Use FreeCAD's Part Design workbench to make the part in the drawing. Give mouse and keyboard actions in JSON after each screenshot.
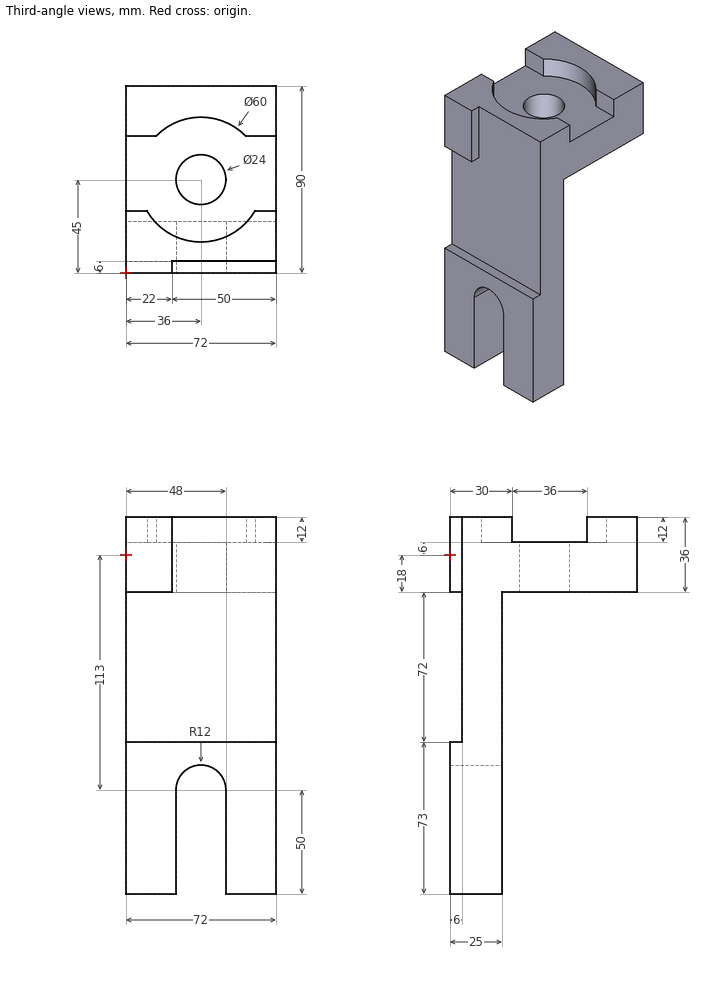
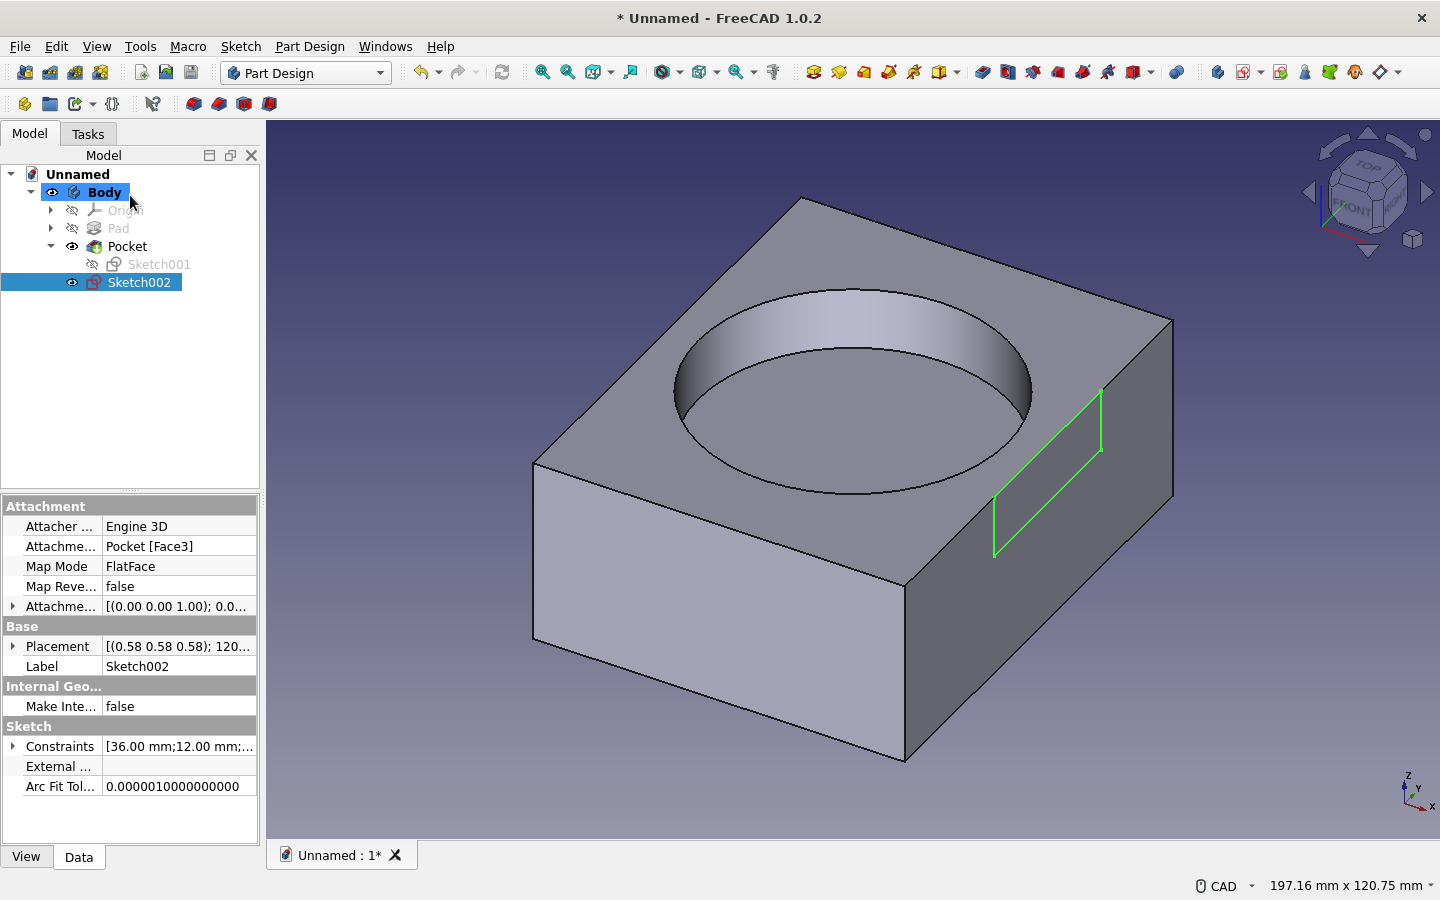
{"action": "left_click", "coordinate": [983, 72]}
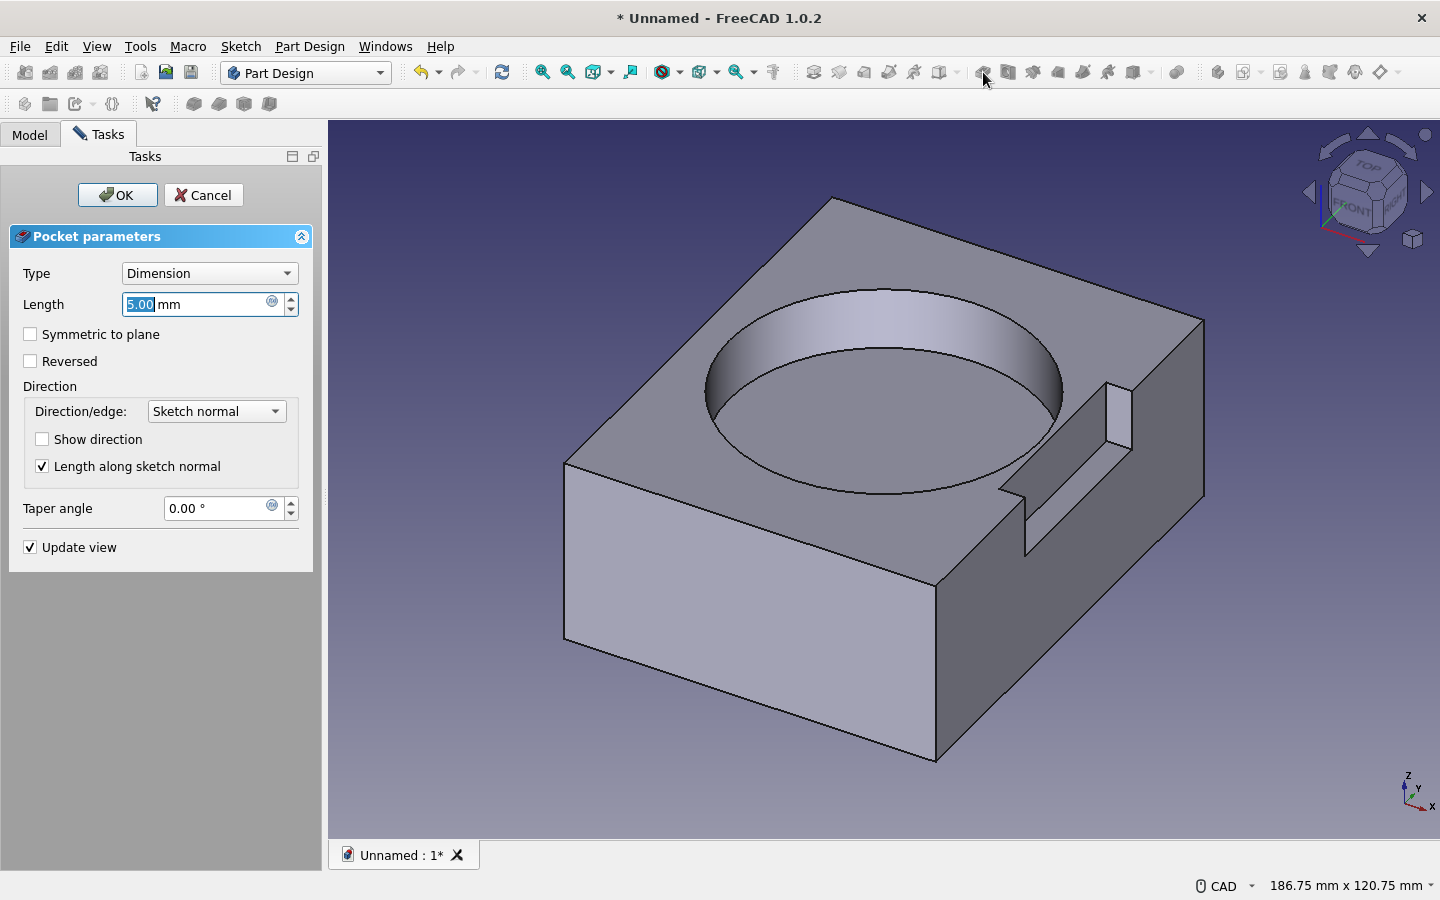
{"action": "left_click", "coordinate": [210, 274]}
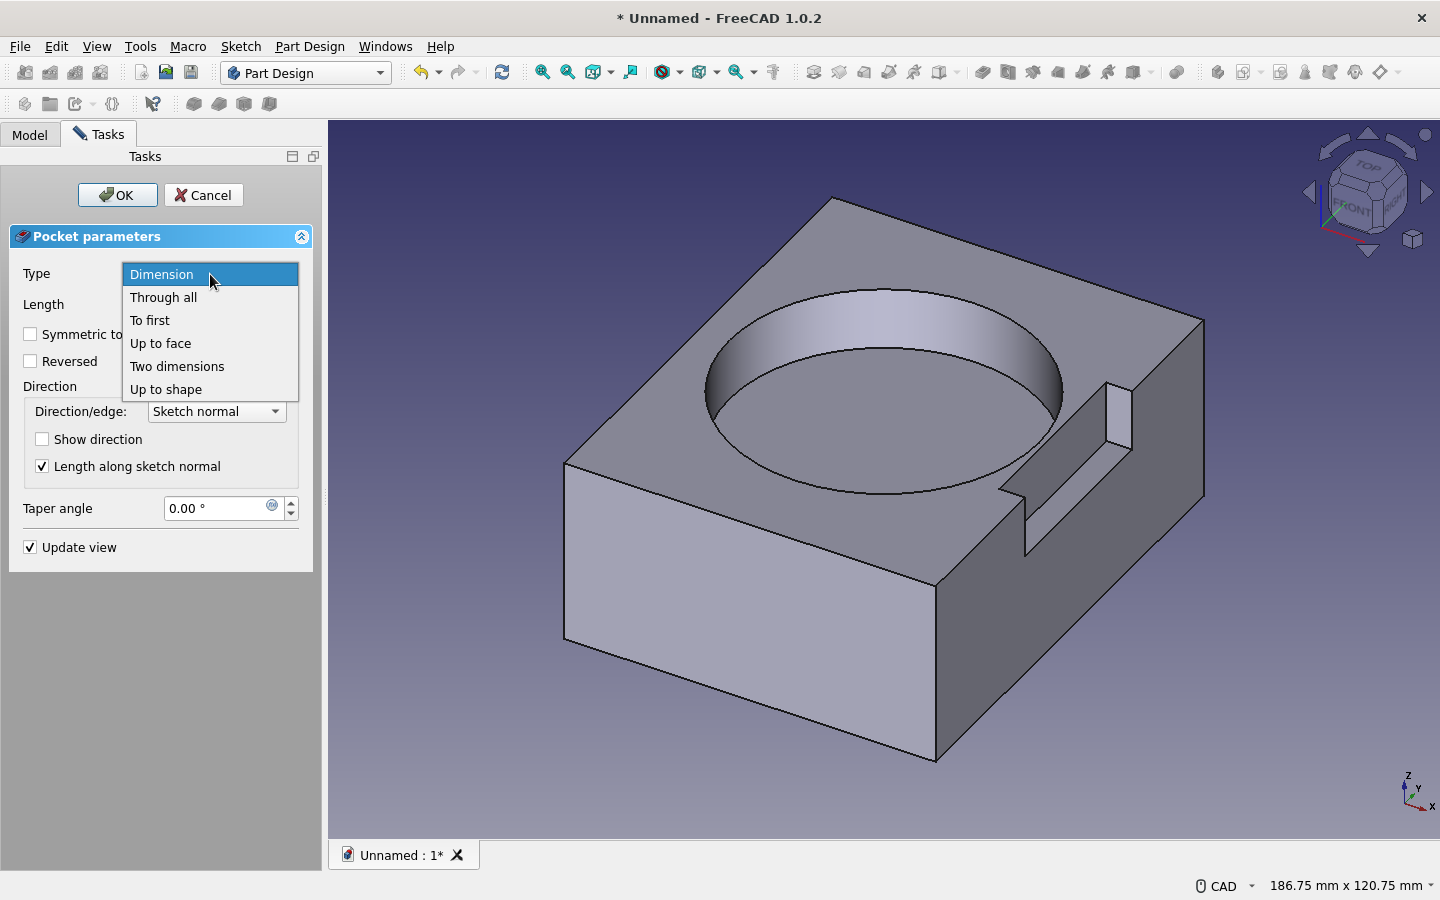
{"action": "left_click", "coordinate": [208, 298]}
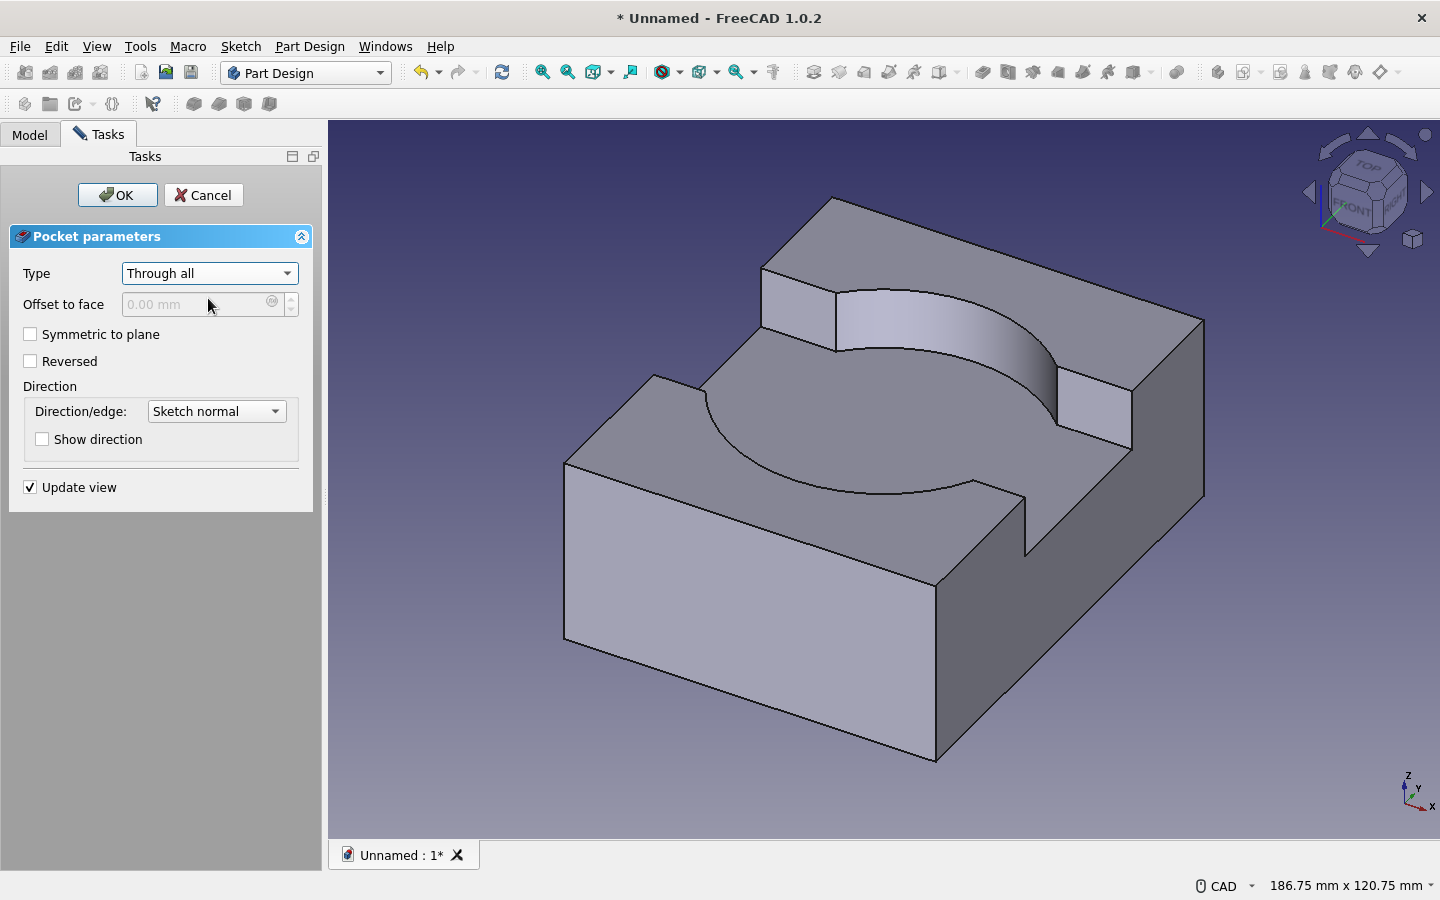
{"action": "left_click", "coordinate": [118, 195]}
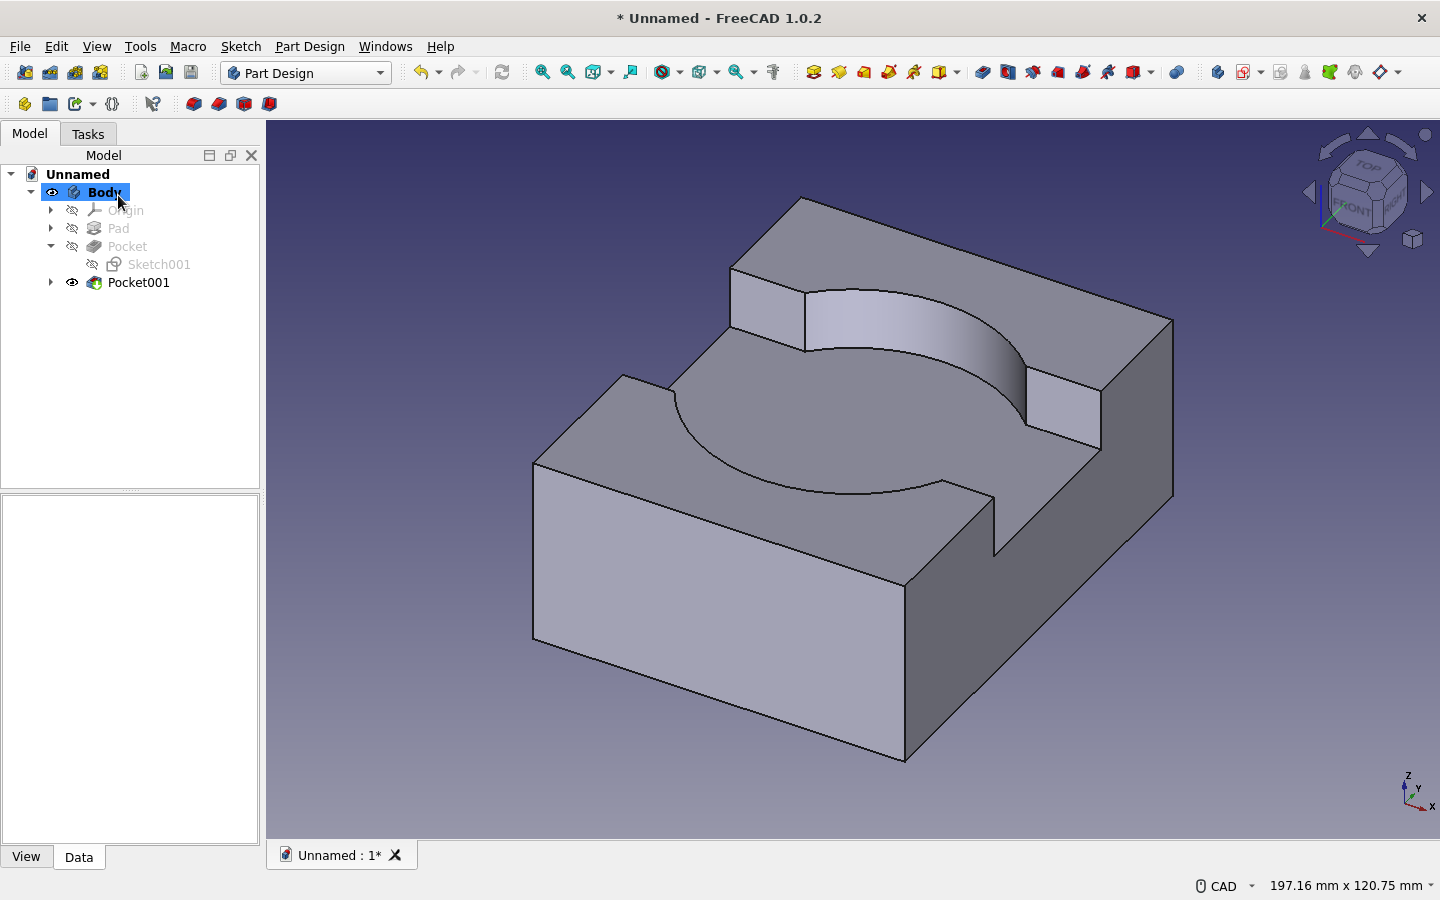
{"action": "left_click", "coordinate": [853, 449]}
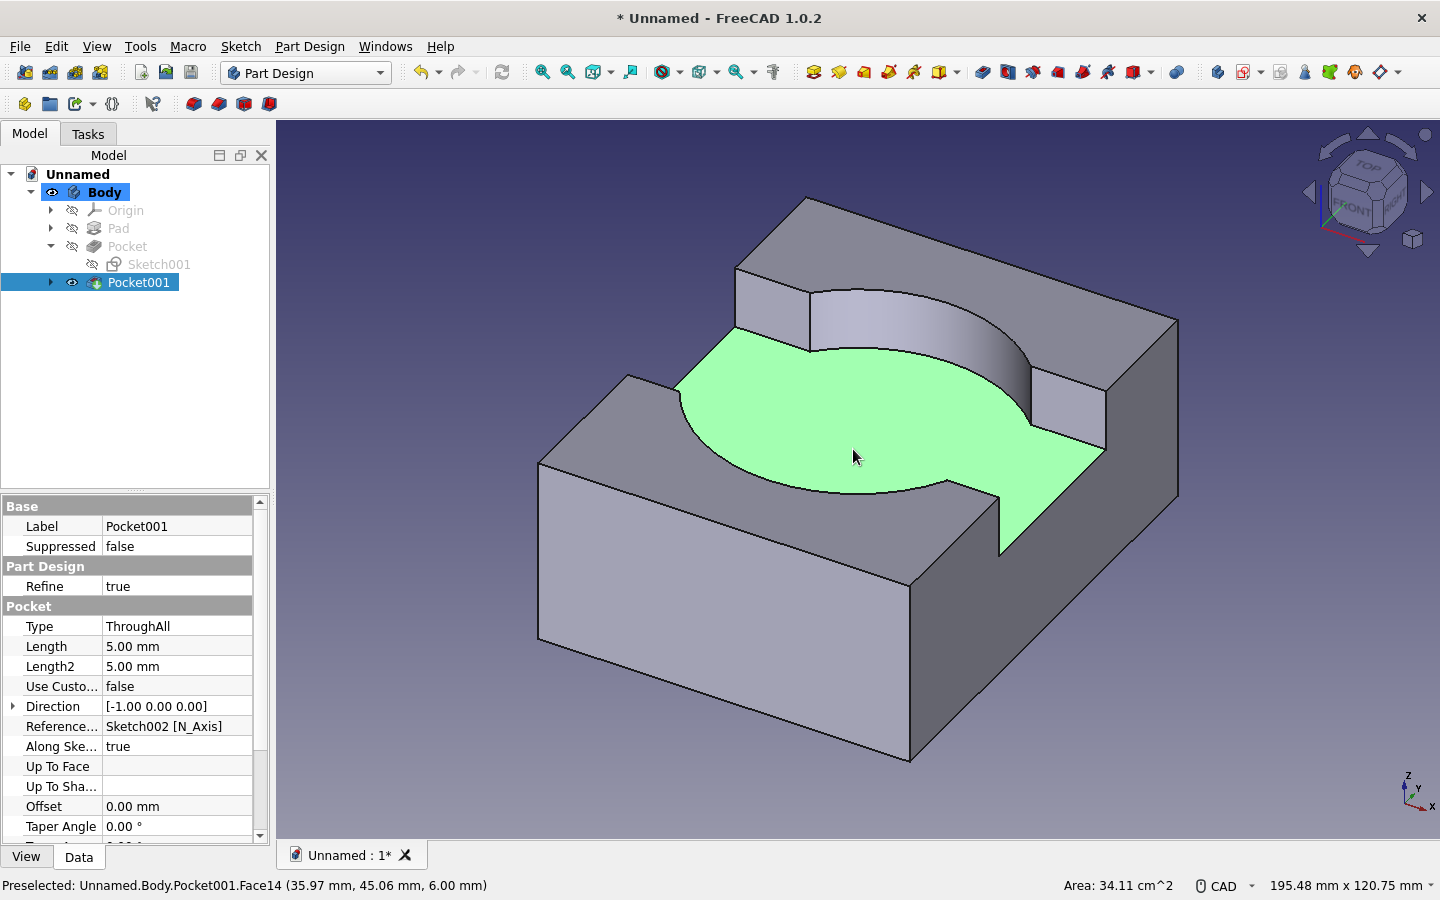
{"action": "left_click", "coordinate": [1242, 72]}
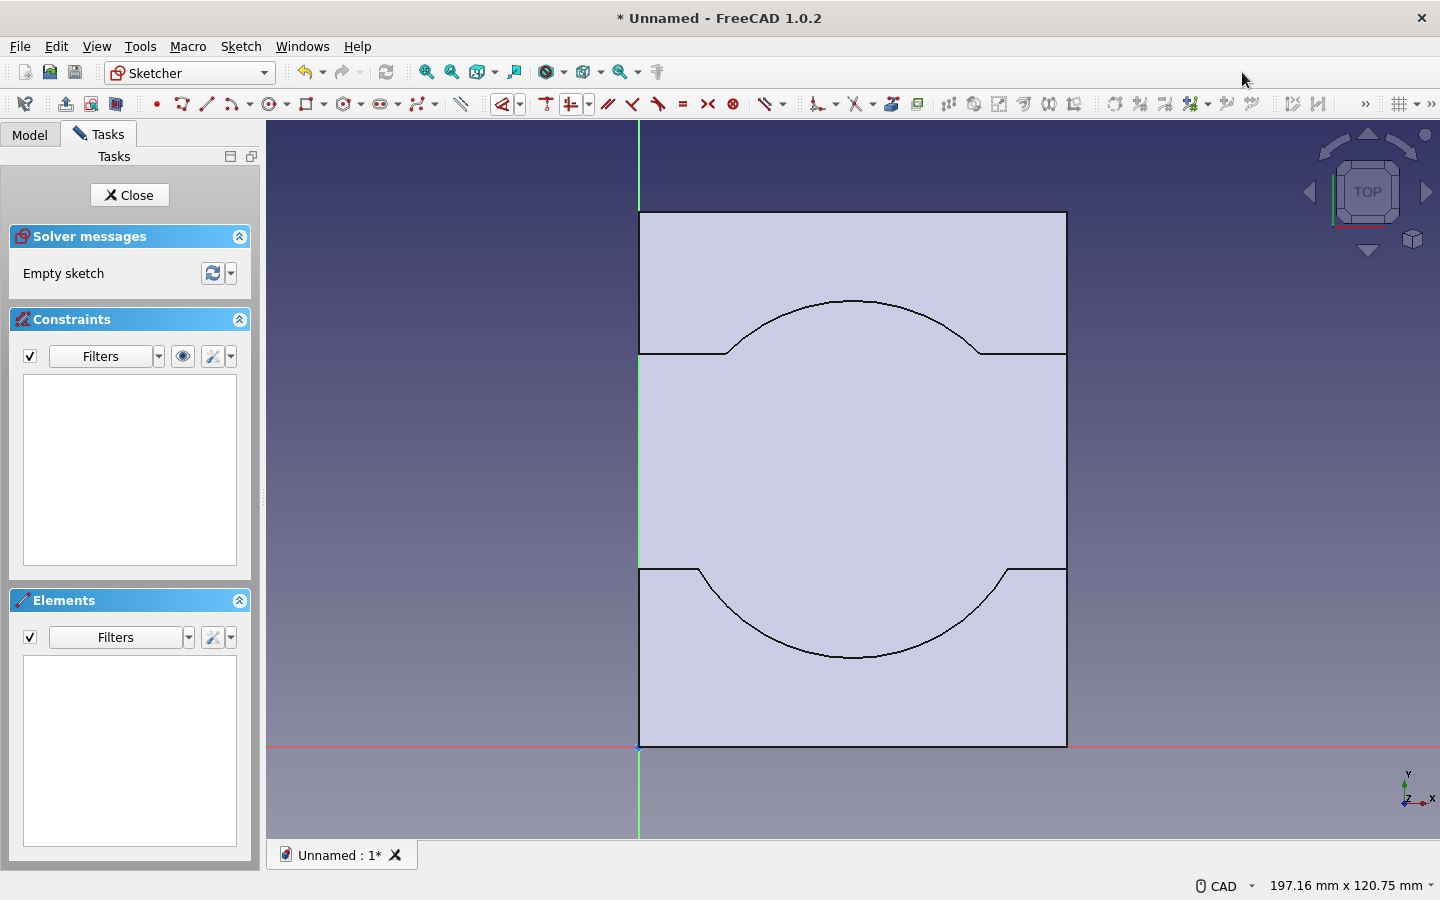
{"action": "key", "text": "q s"}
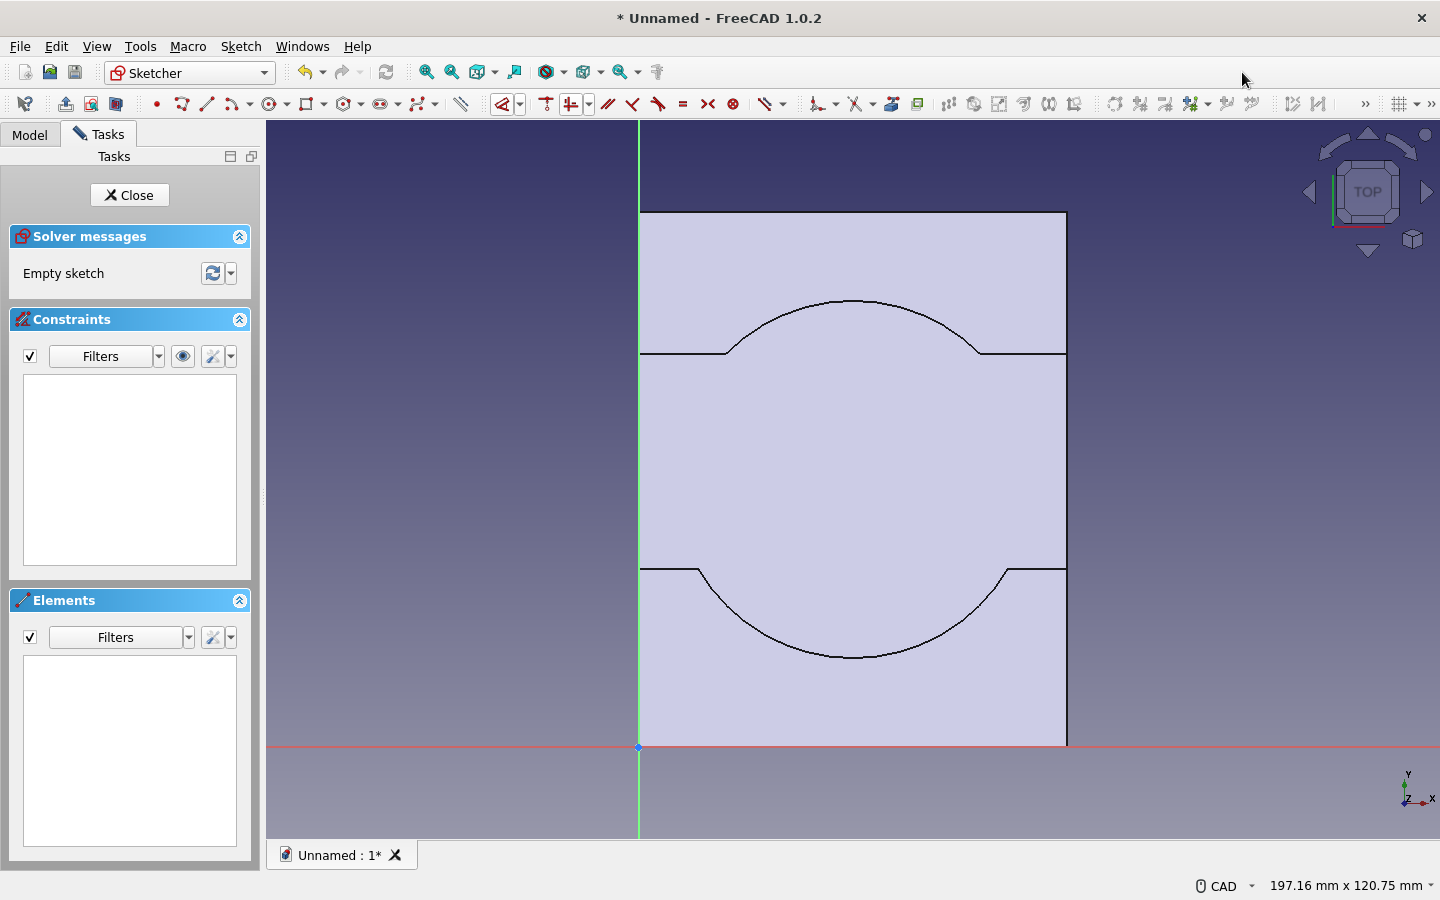
{"action": "scroll", "coordinate": [776, 778], "scroll_direction": "up", "scroll_amount": 2}